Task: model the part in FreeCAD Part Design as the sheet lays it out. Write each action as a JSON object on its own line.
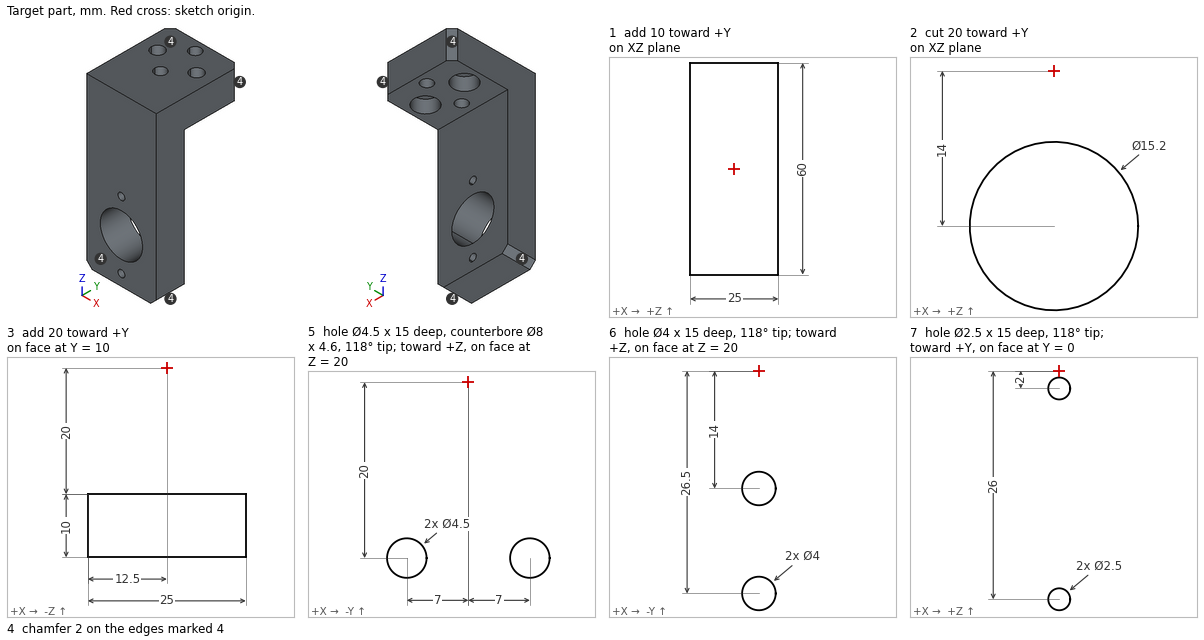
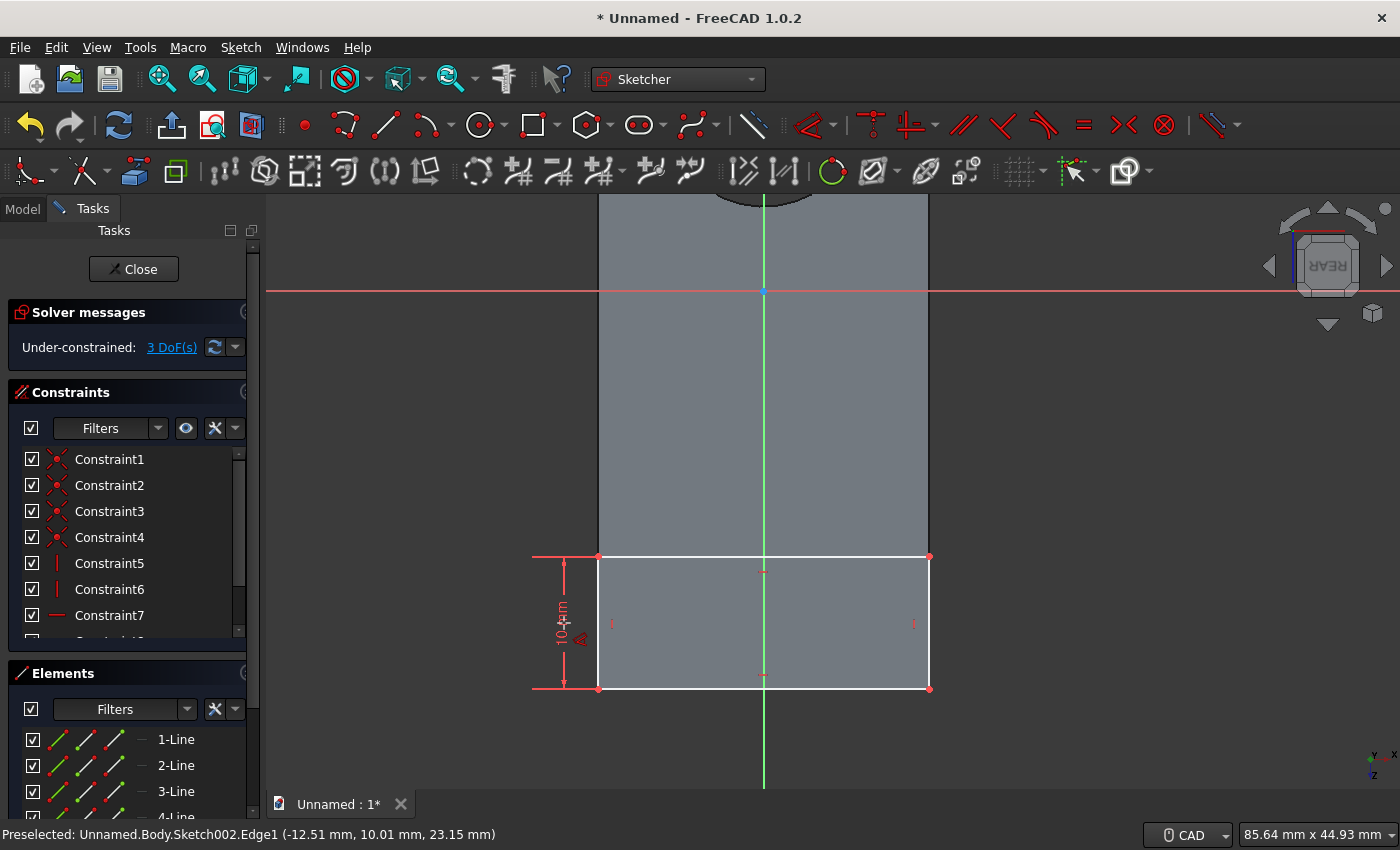
{"action": "left_click", "coordinate": [697, 689]}
{"action": "left_click", "coordinate": [687, 723]}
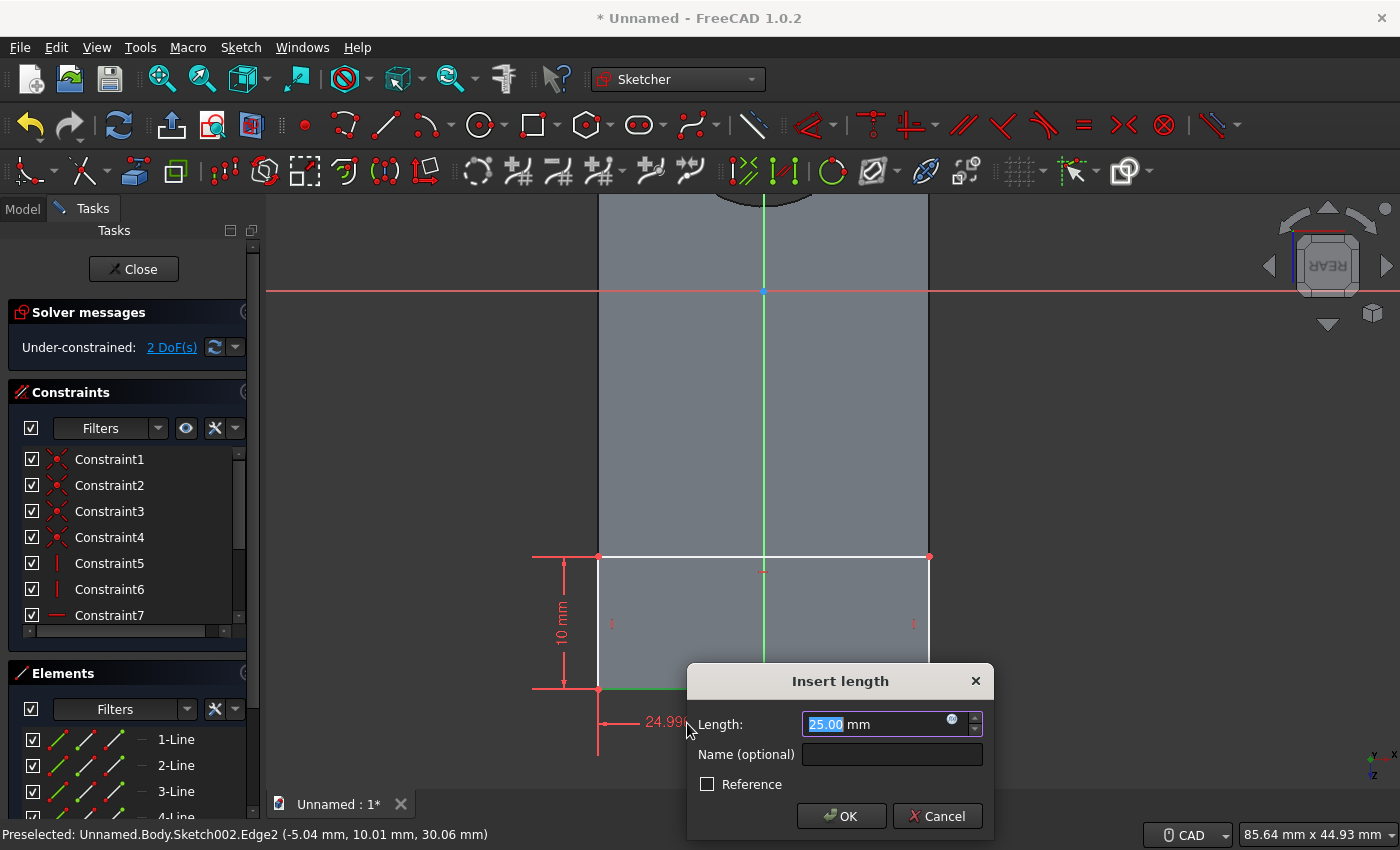
{"action": "type", "text": "25"}
{"action": "key", "text": "Return"}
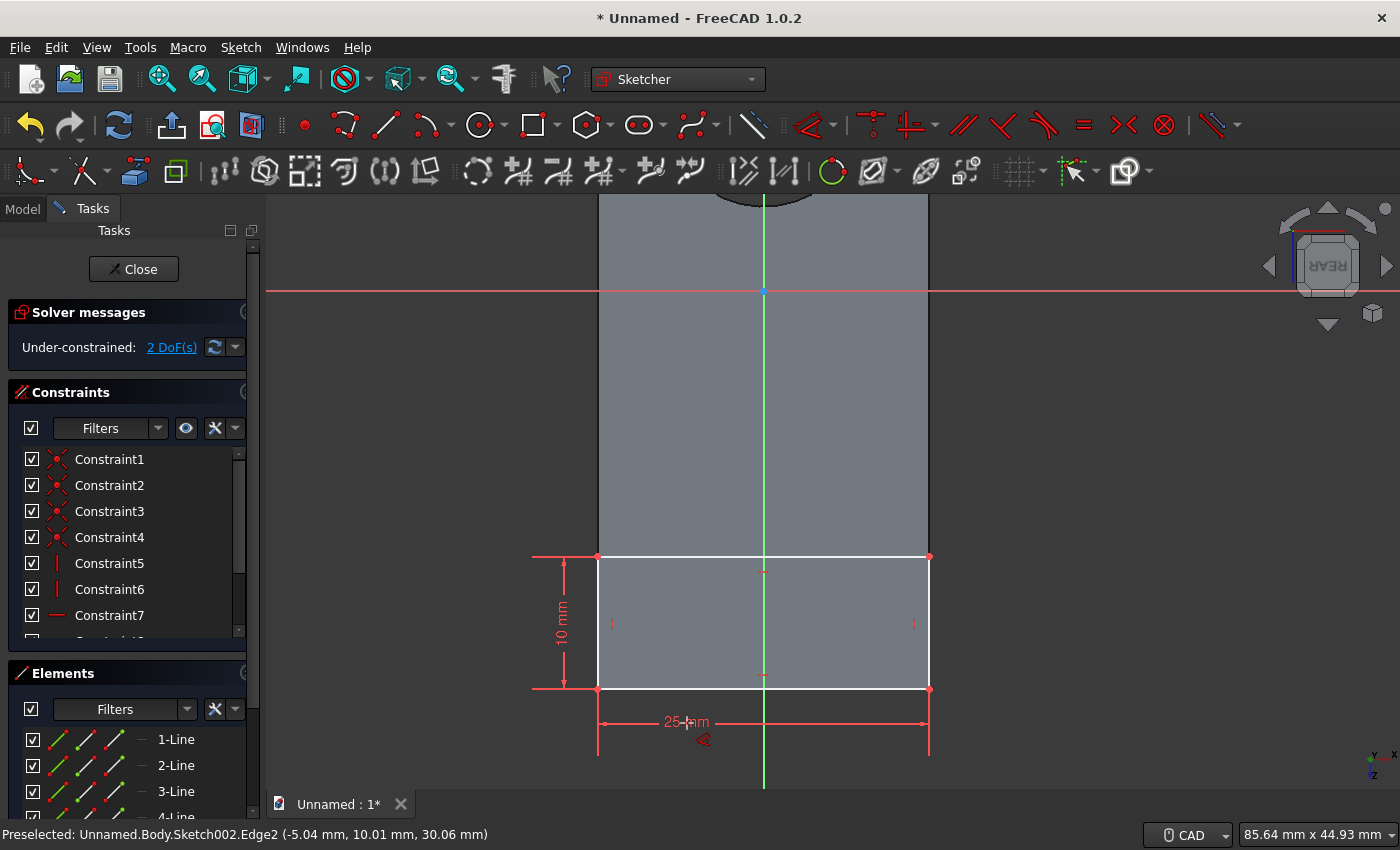
{"action": "left_click", "coordinate": [598, 557]}
{"action": "left_click", "coordinate": [564, 424]}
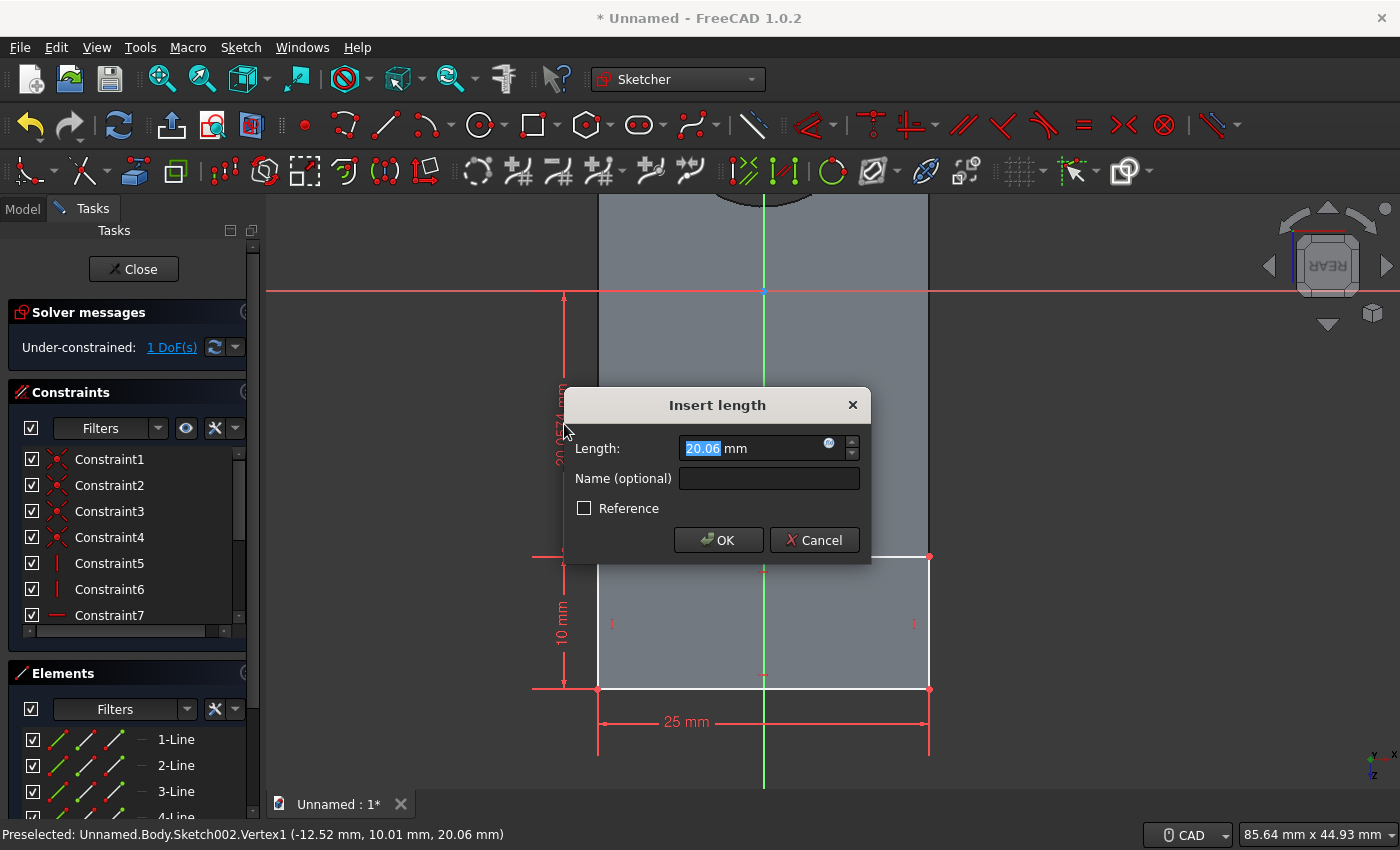
{"action": "type", "text": "20"}
{"action": "key", "text": "Return"}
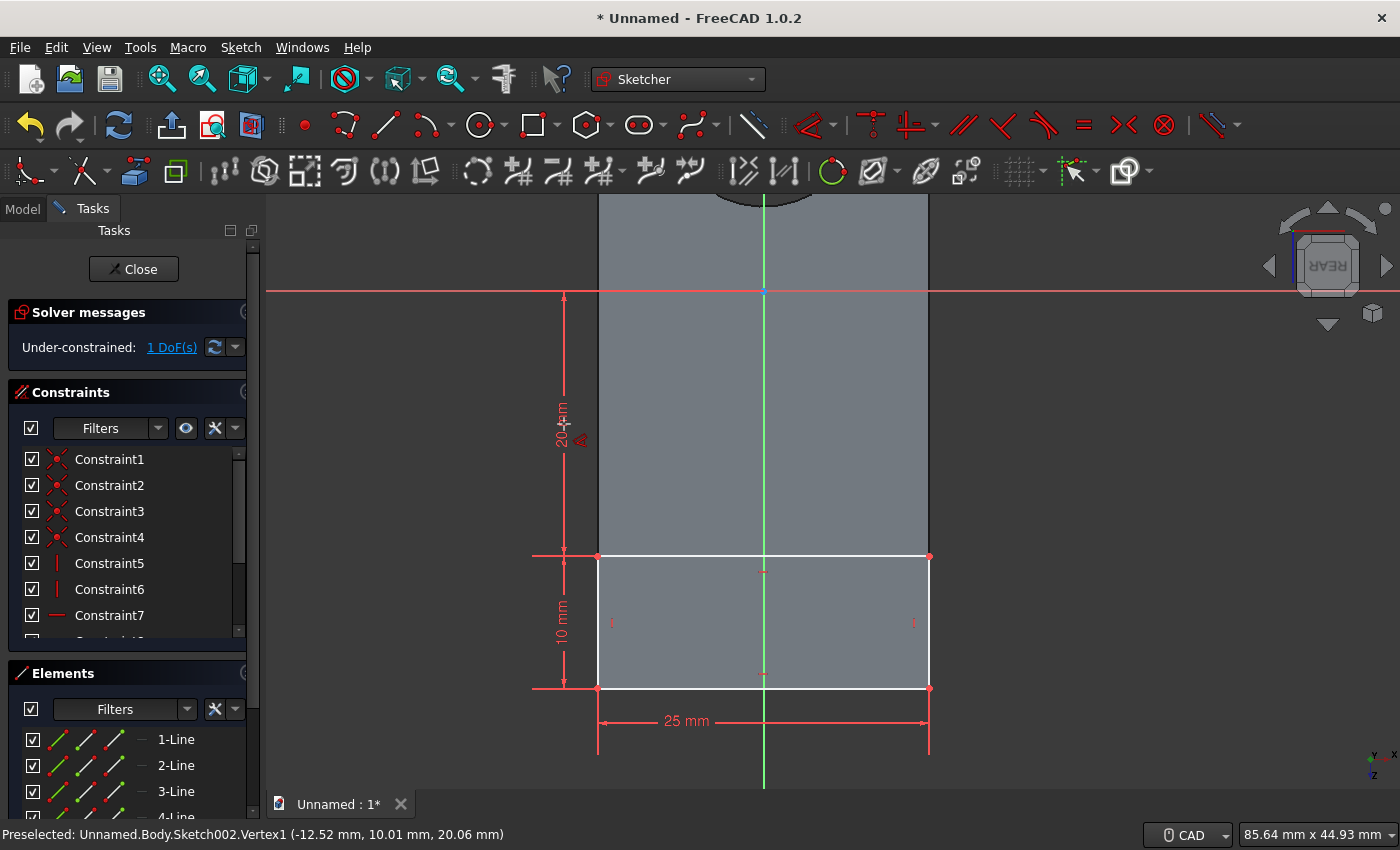
{"action": "left_click", "coordinate": [598, 556]}
{"action": "left_click", "coordinate": [681, 257]}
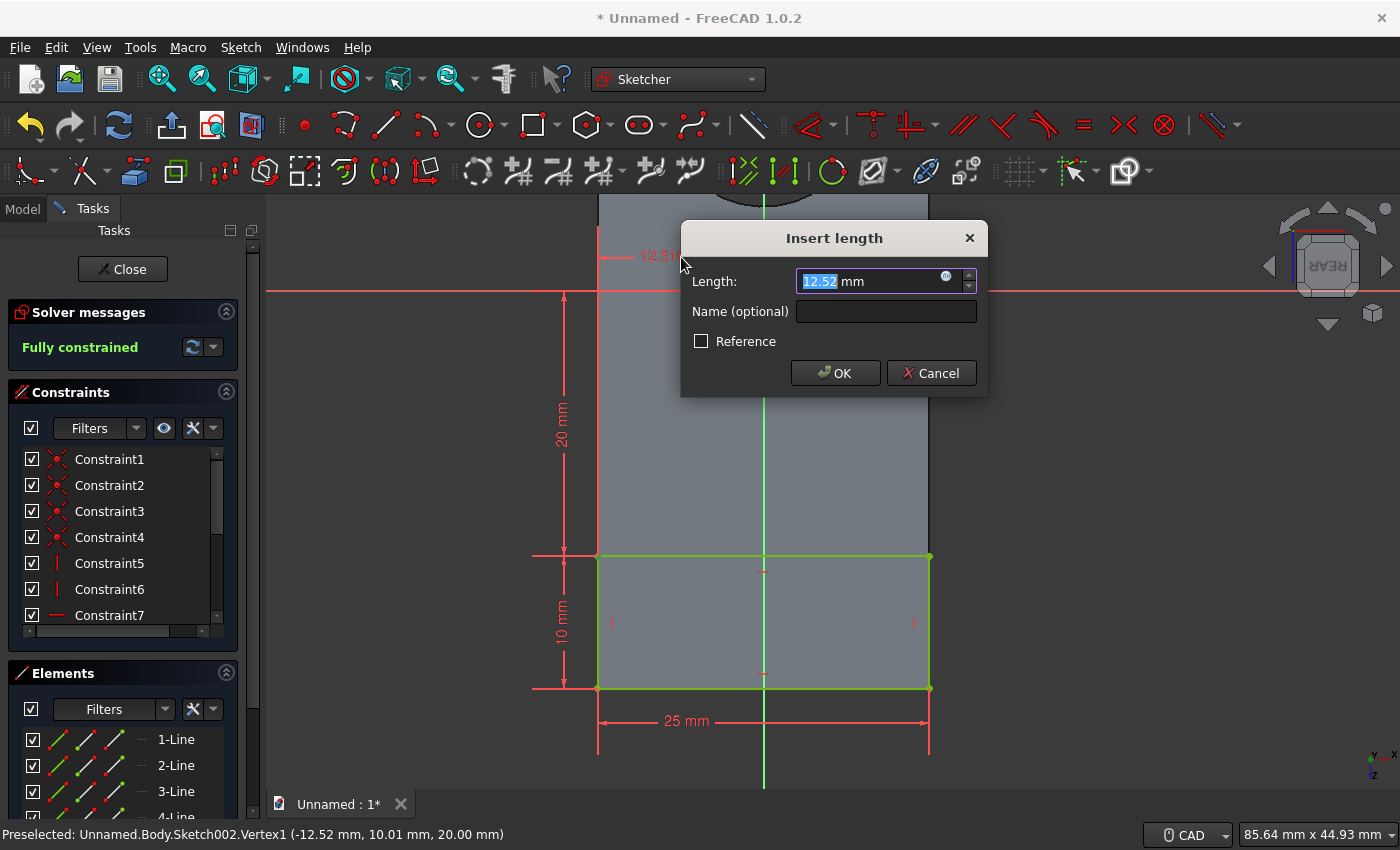
{"action": "type", "text": "12.5"}
{"action": "key", "text": "Return"}
{"action": "key", "text": "Escape"}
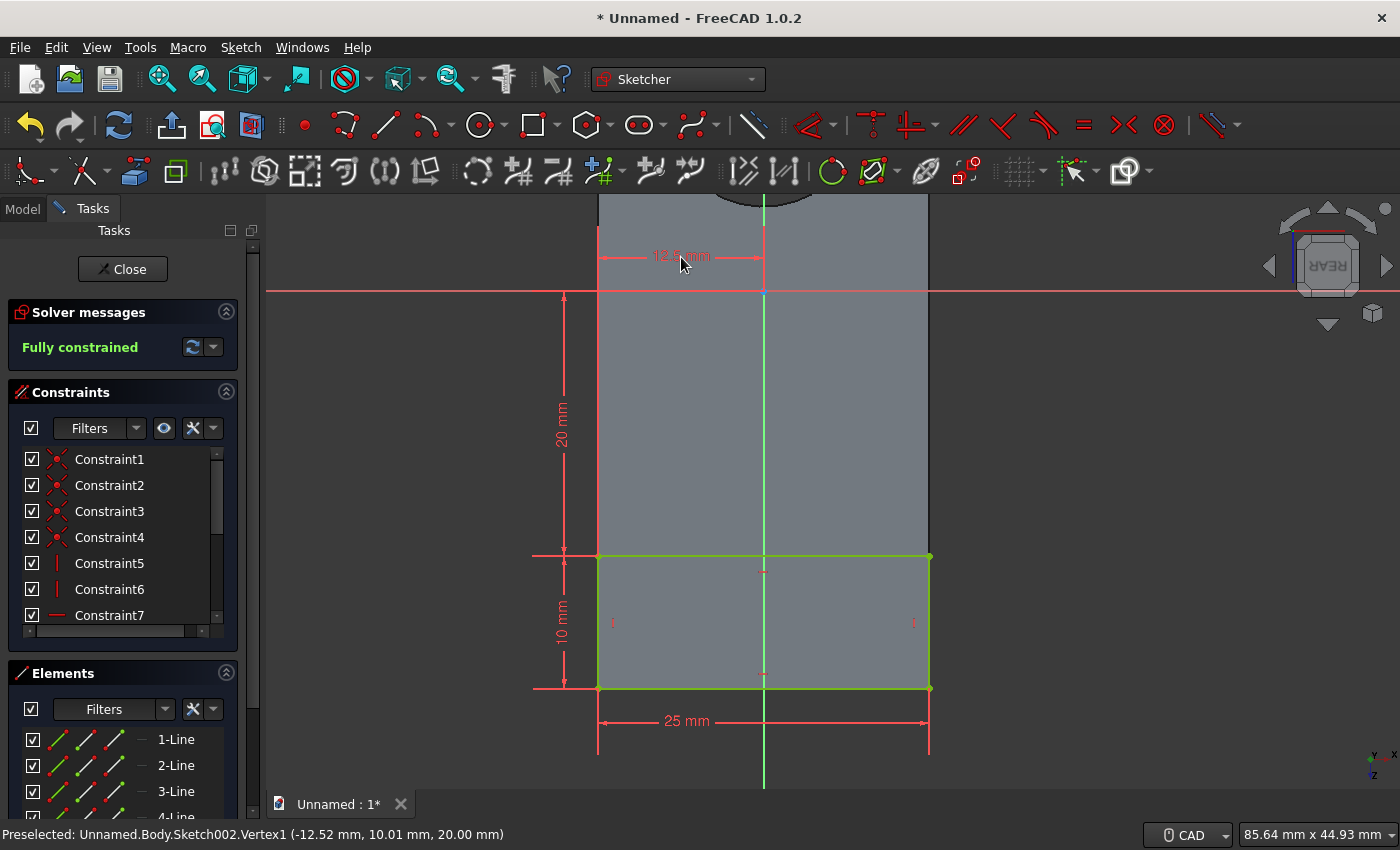
{"action": "left_click", "coordinate": [123, 269]}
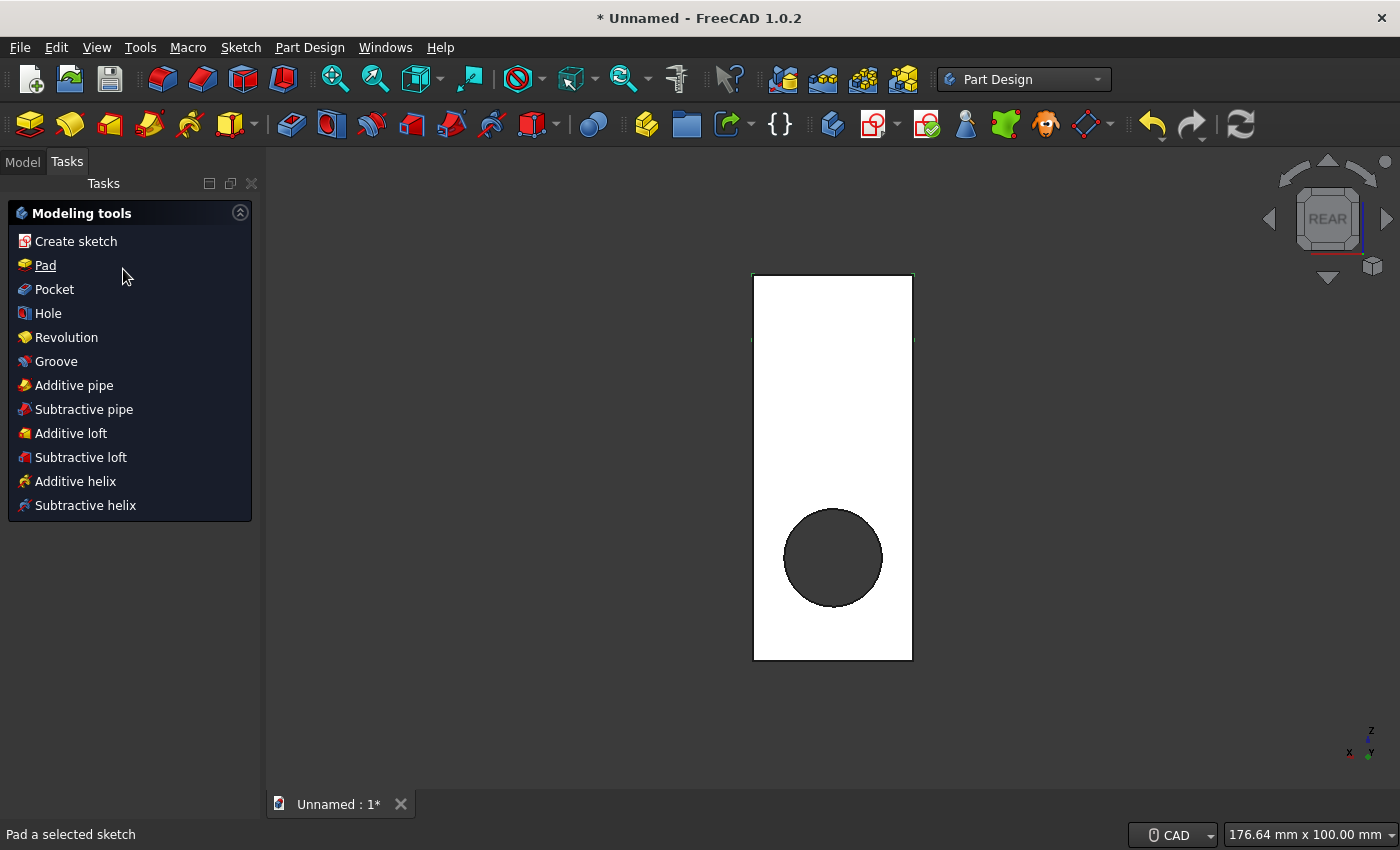
{"action": "left_click", "coordinate": [30, 124]}